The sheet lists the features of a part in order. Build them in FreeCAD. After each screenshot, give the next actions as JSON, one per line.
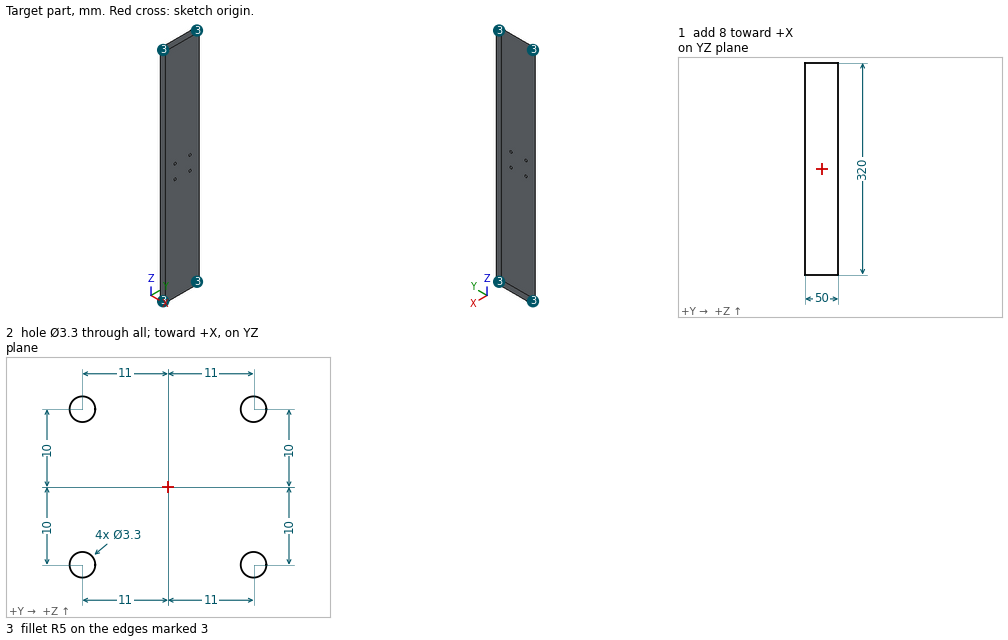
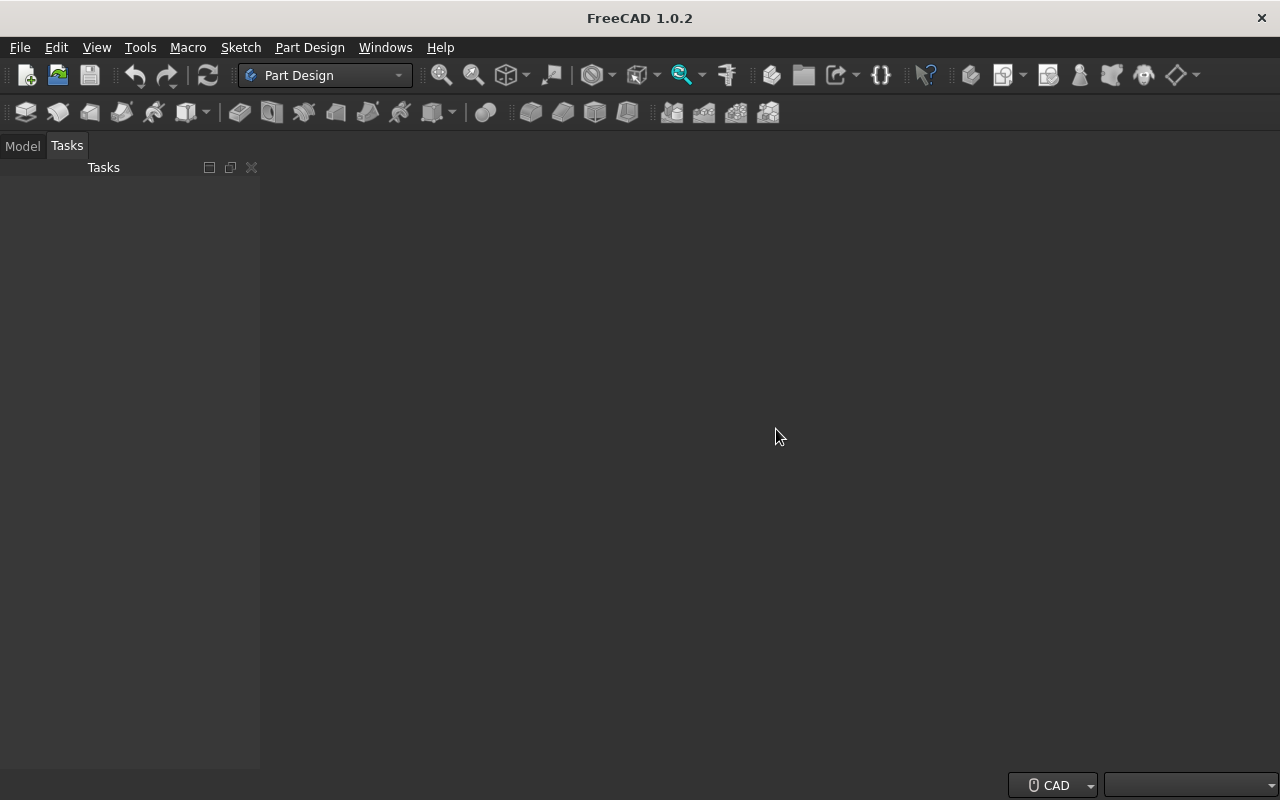
{"action": "left_click", "coordinate": [26, 76]}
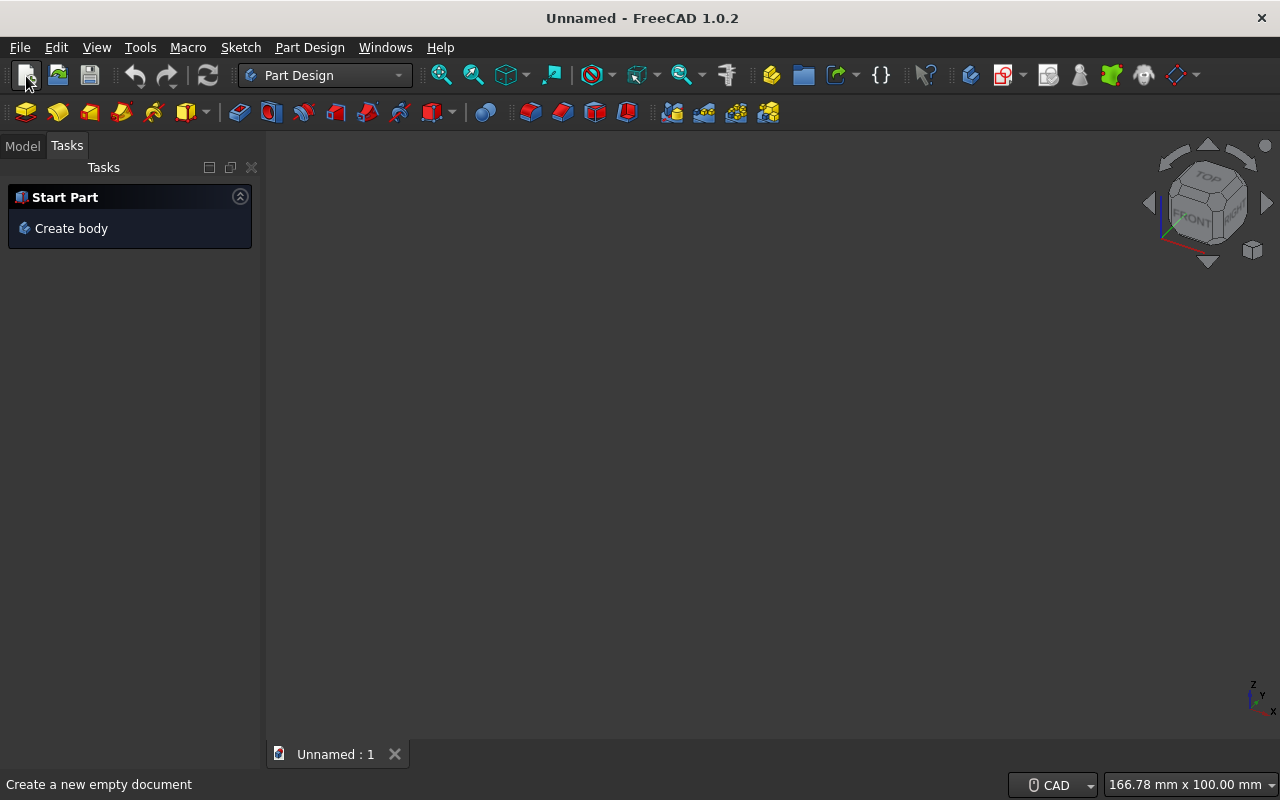
{"action": "left_click", "coordinate": [1004, 76]}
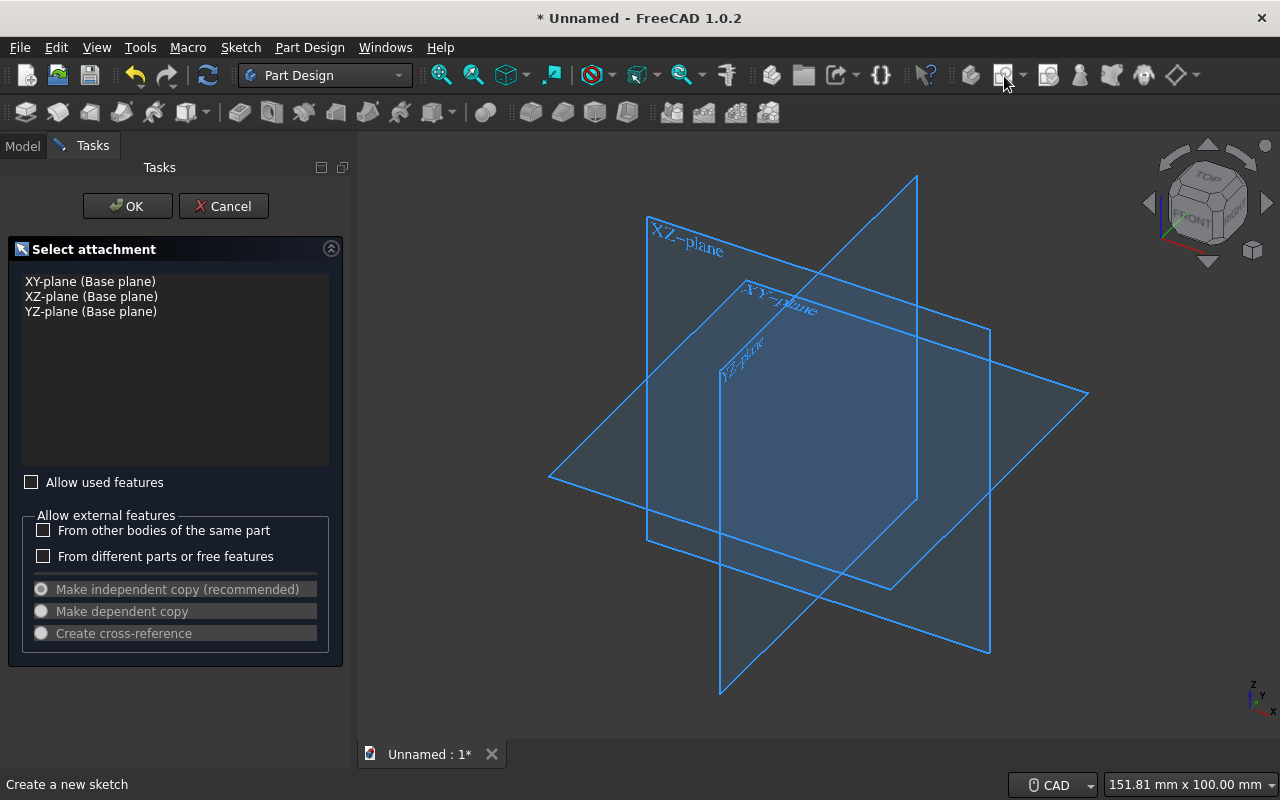
{"action": "left_click", "coordinate": [82, 312]}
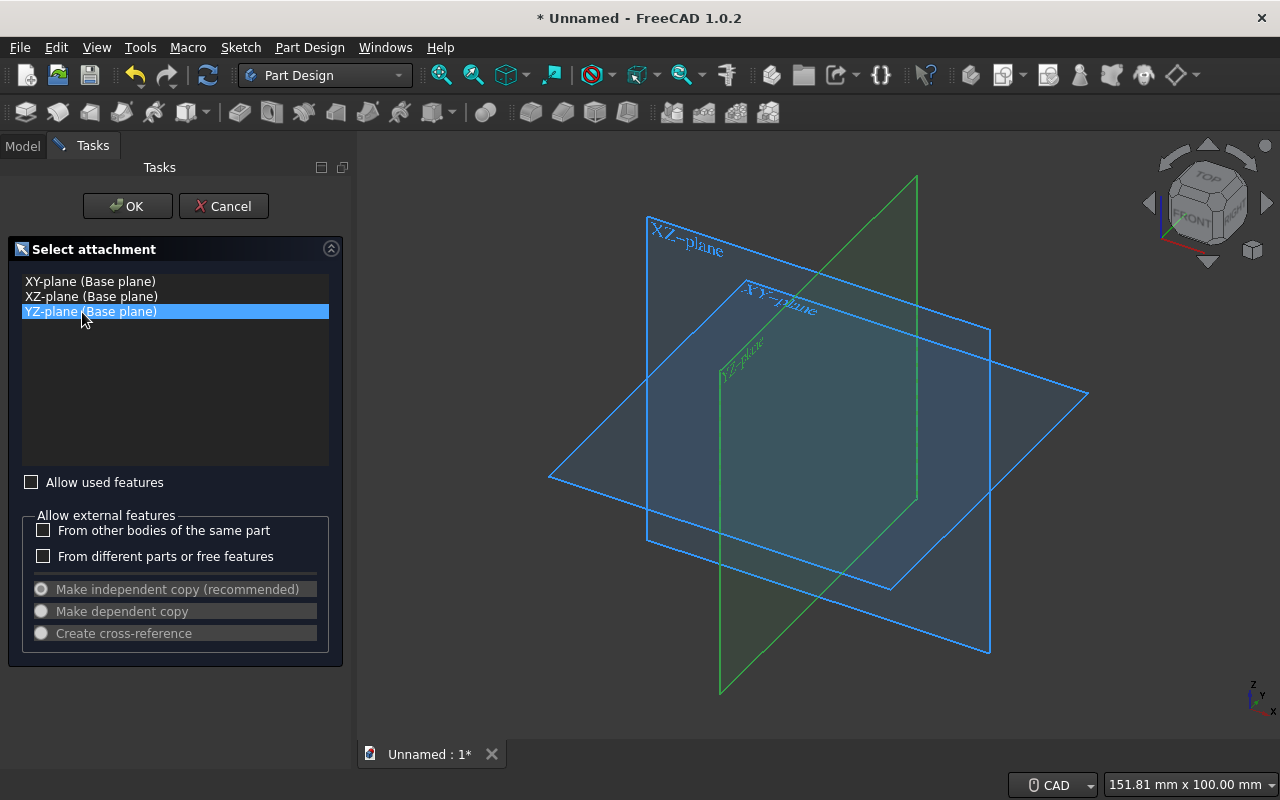
{"action": "left_click", "coordinate": [128, 206]}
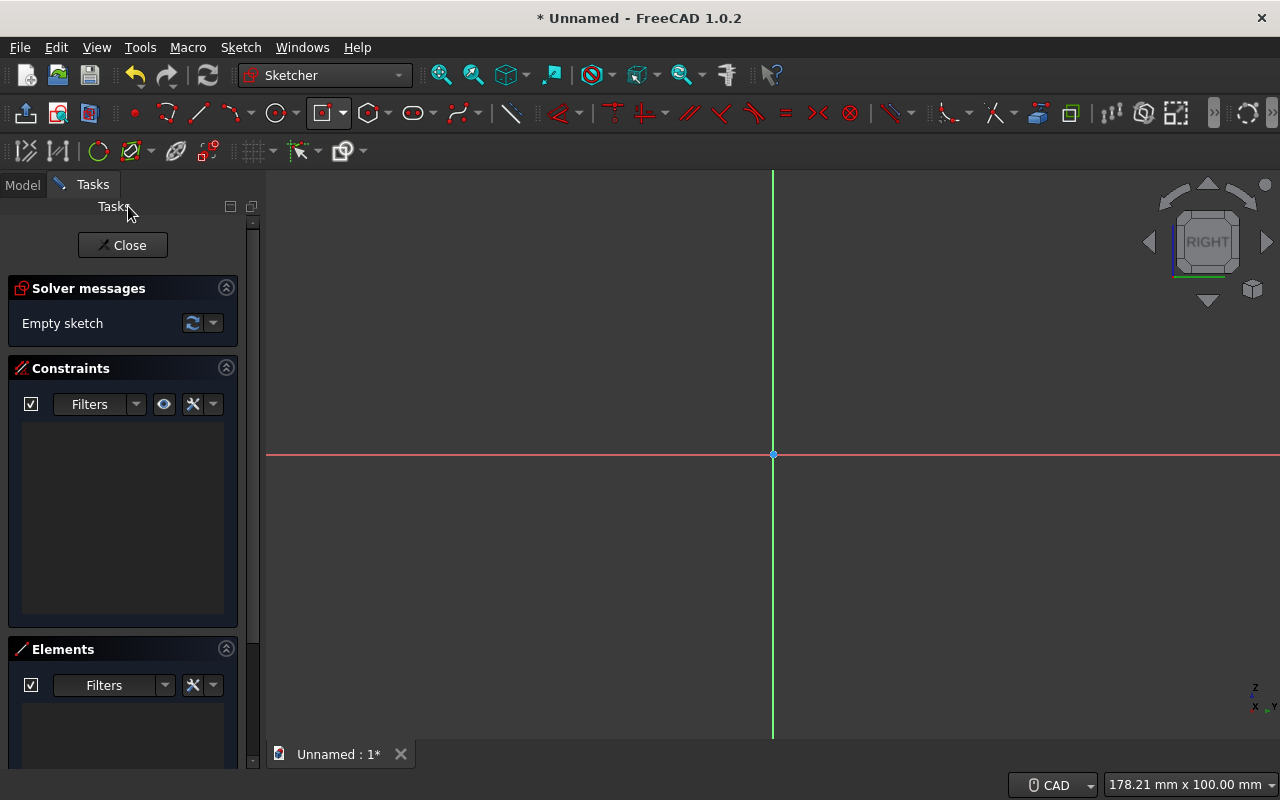
{"action": "scroll", "coordinate": [687, 454], "scroll_direction": "down", "scroll_amount": 8}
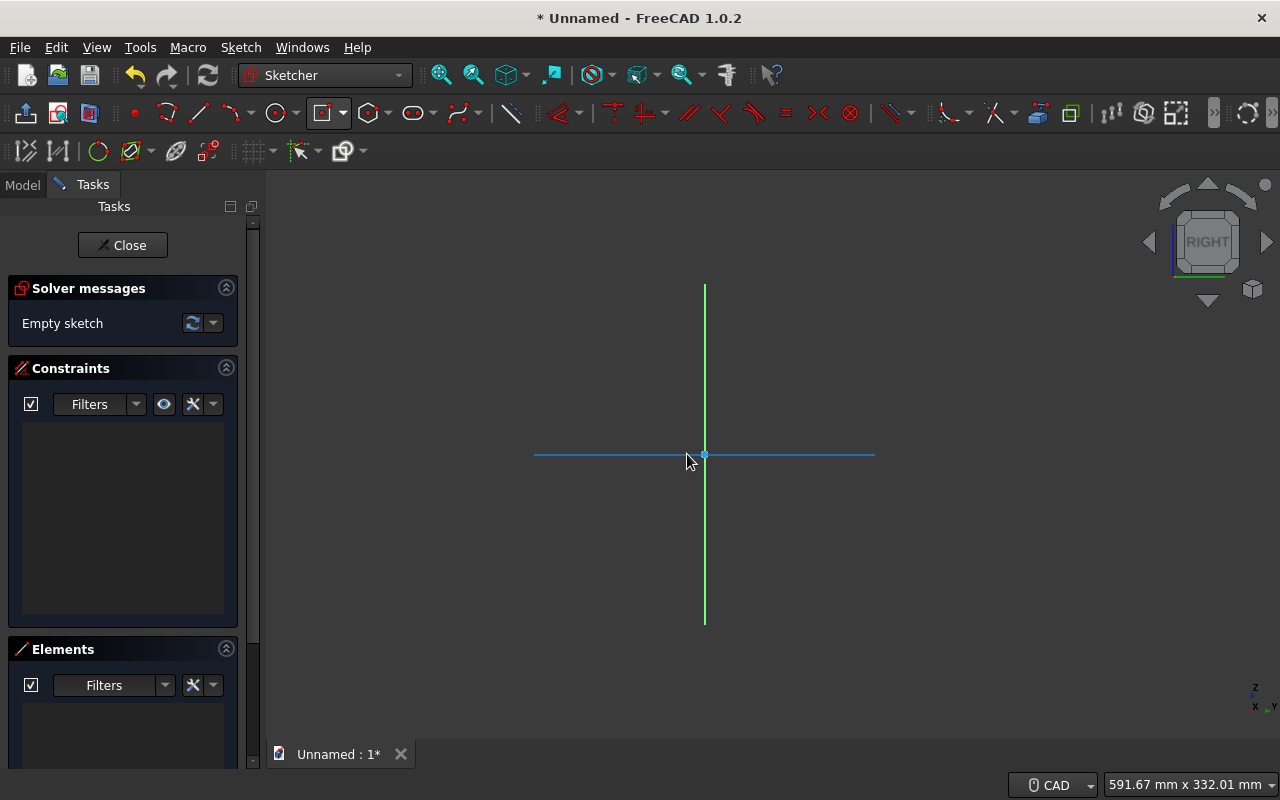
{"action": "left_click", "coordinate": [322, 114]}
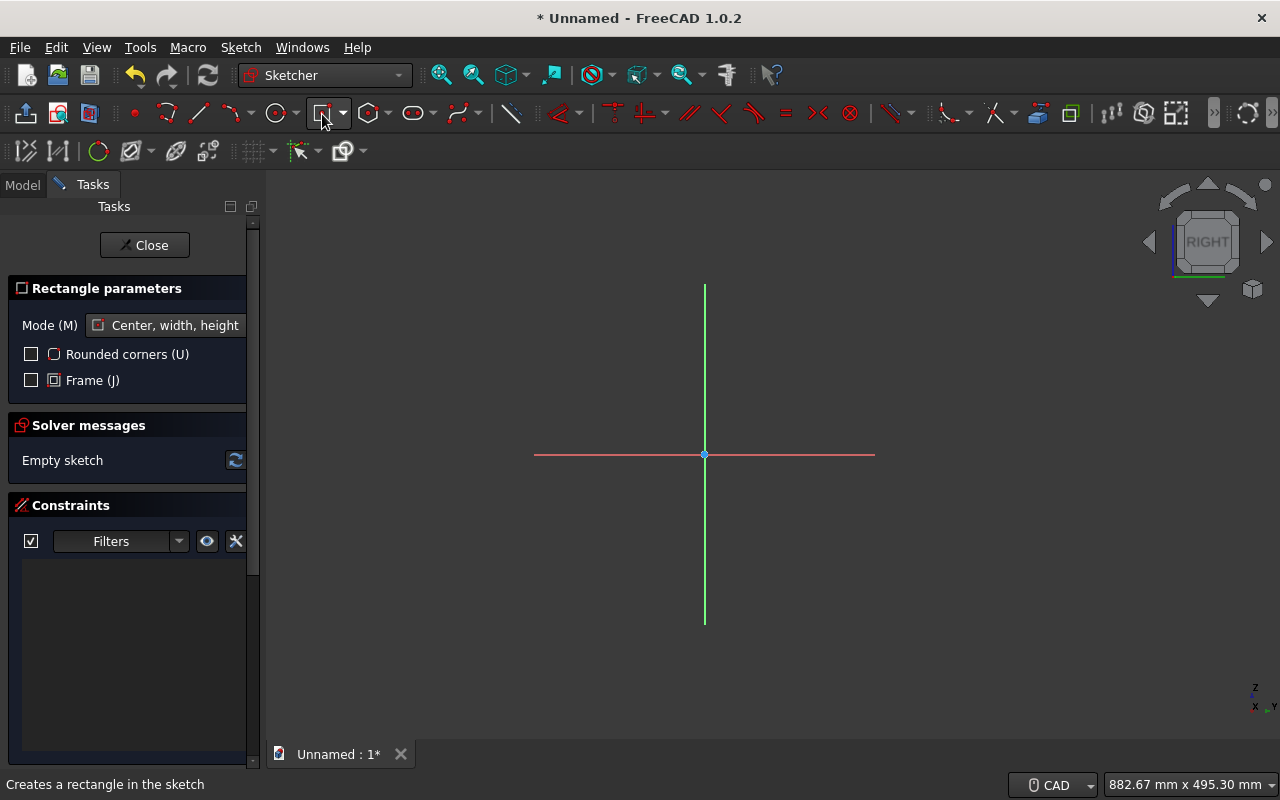
{"action": "left_click", "coordinate": [705, 454]}
{"action": "left_click", "coordinate": [733, 271]}
{"action": "key", "text": "Escape"}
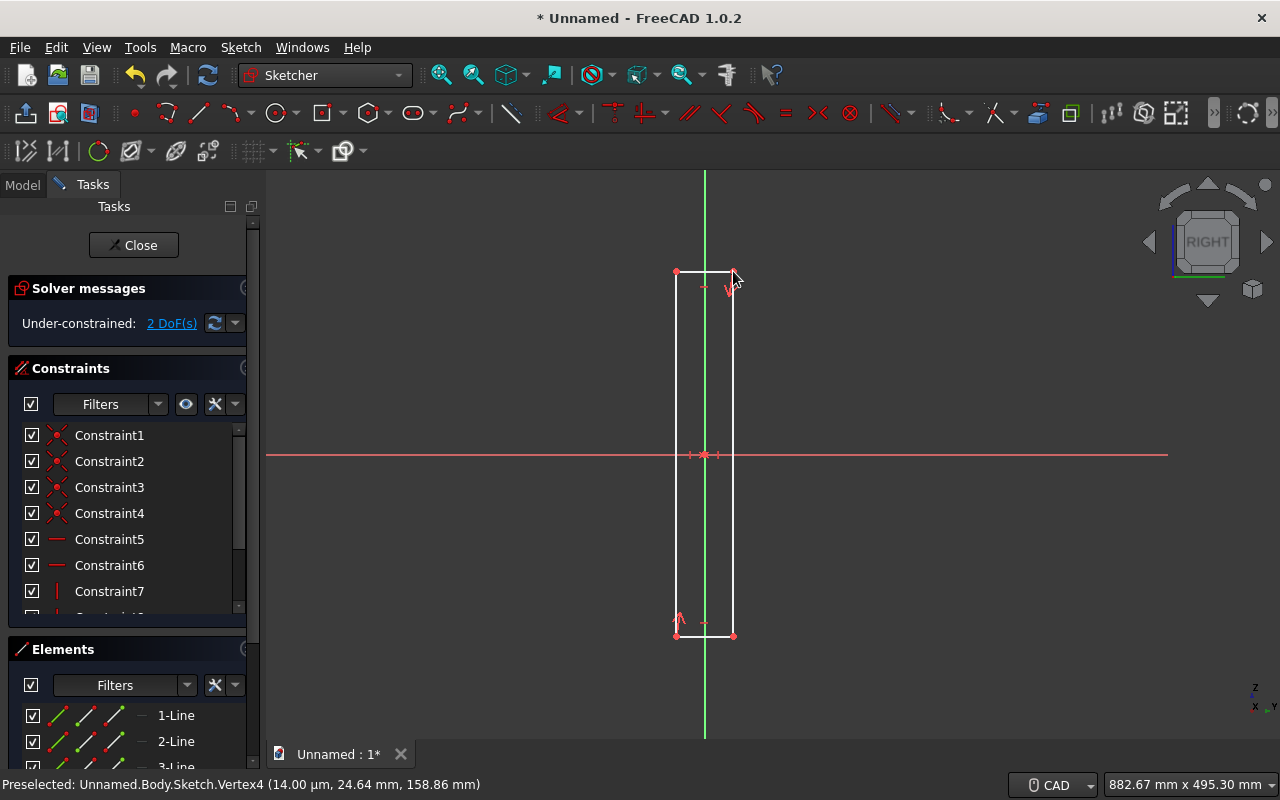
{"action": "key", "text": "d"}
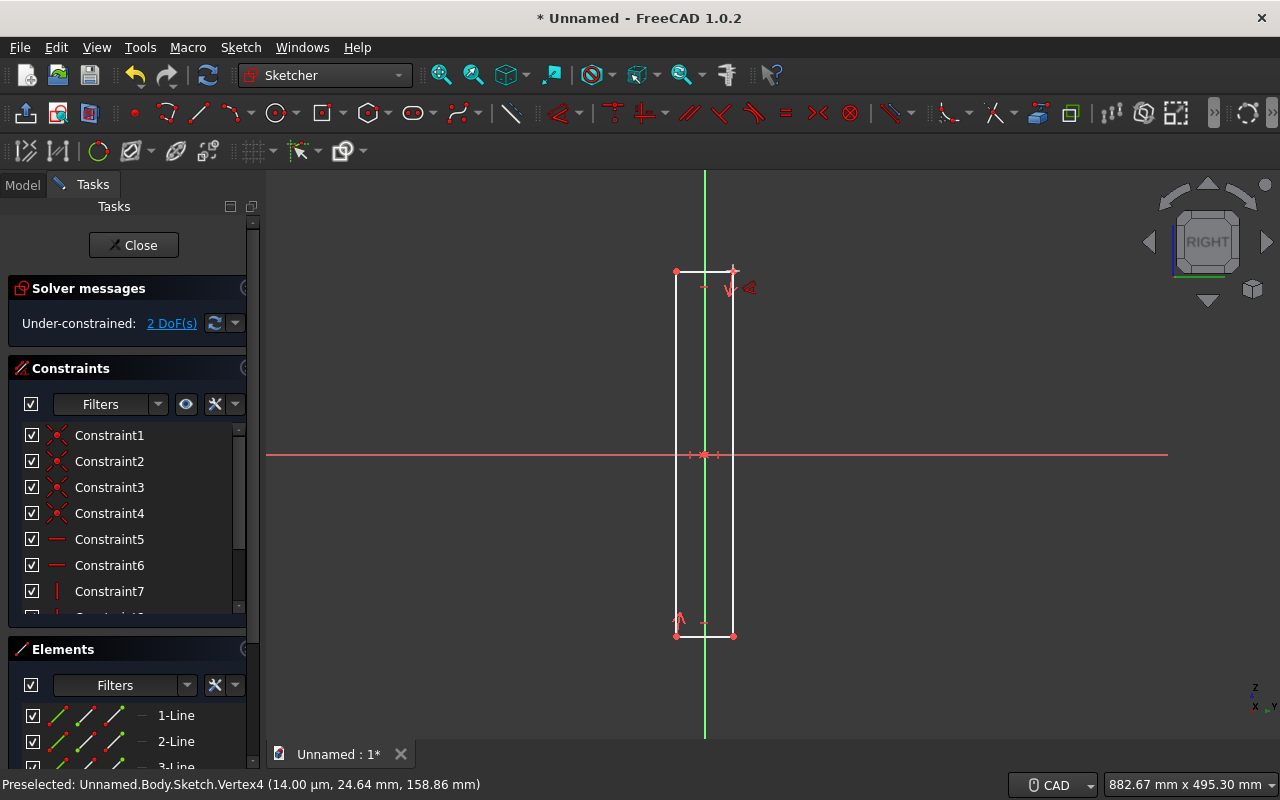
{"action": "left_click", "coordinate": [693, 637]}
{"action": "left_click", "coordinate": [692, 671]}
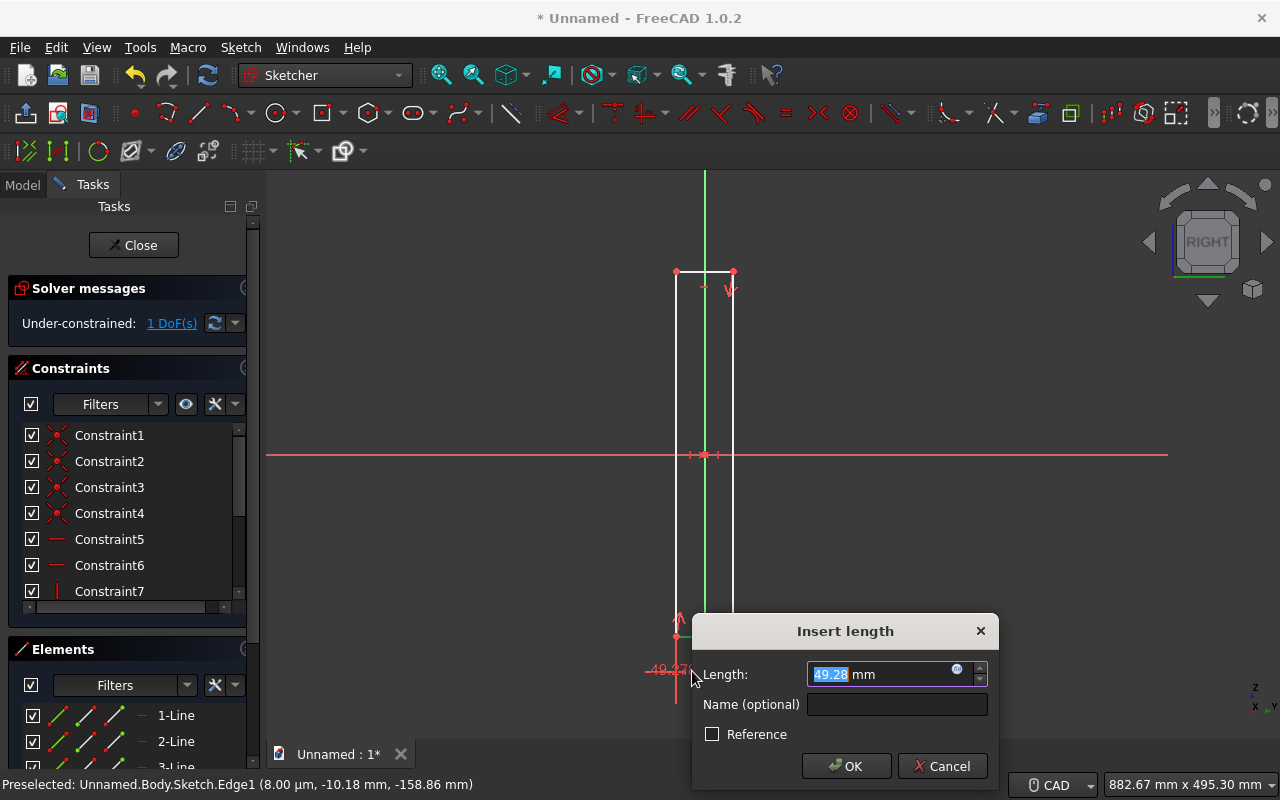
{"action": "type", "text": "50"}
{"action": "key", "text": "Return"}